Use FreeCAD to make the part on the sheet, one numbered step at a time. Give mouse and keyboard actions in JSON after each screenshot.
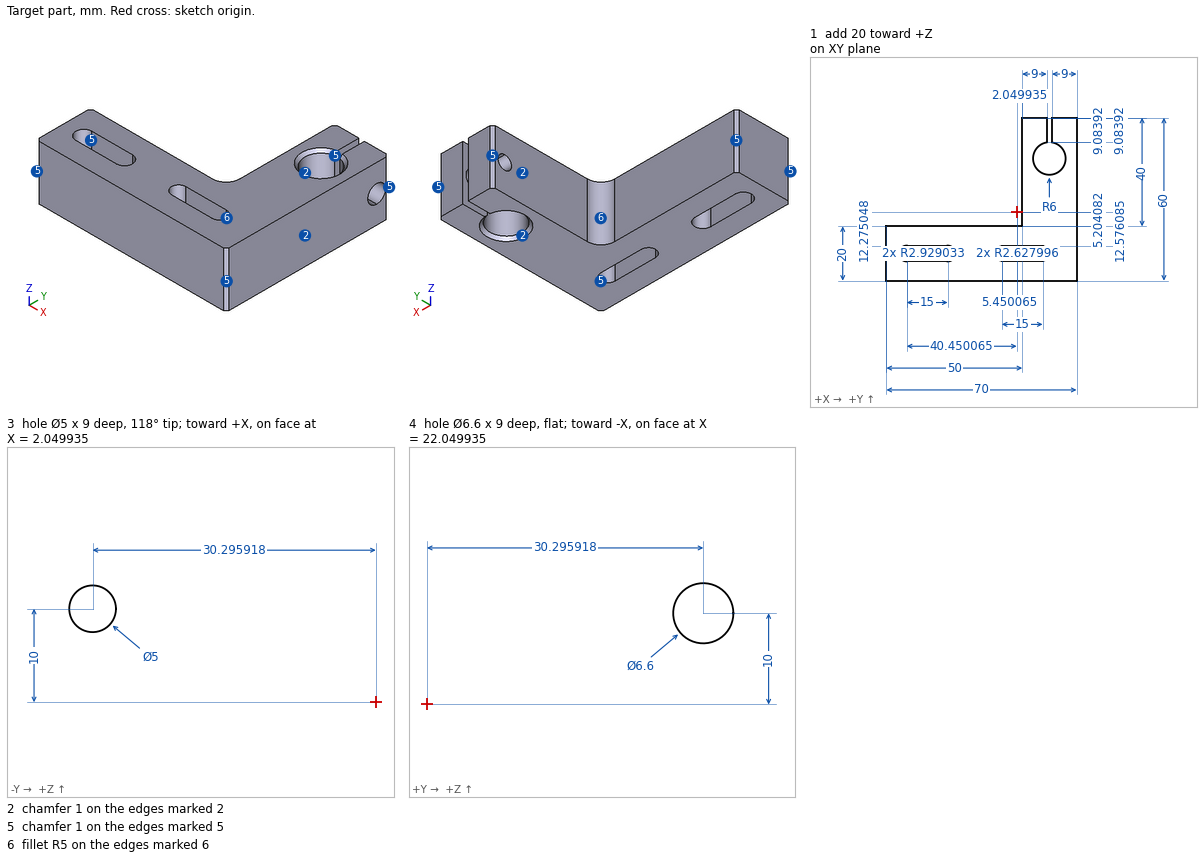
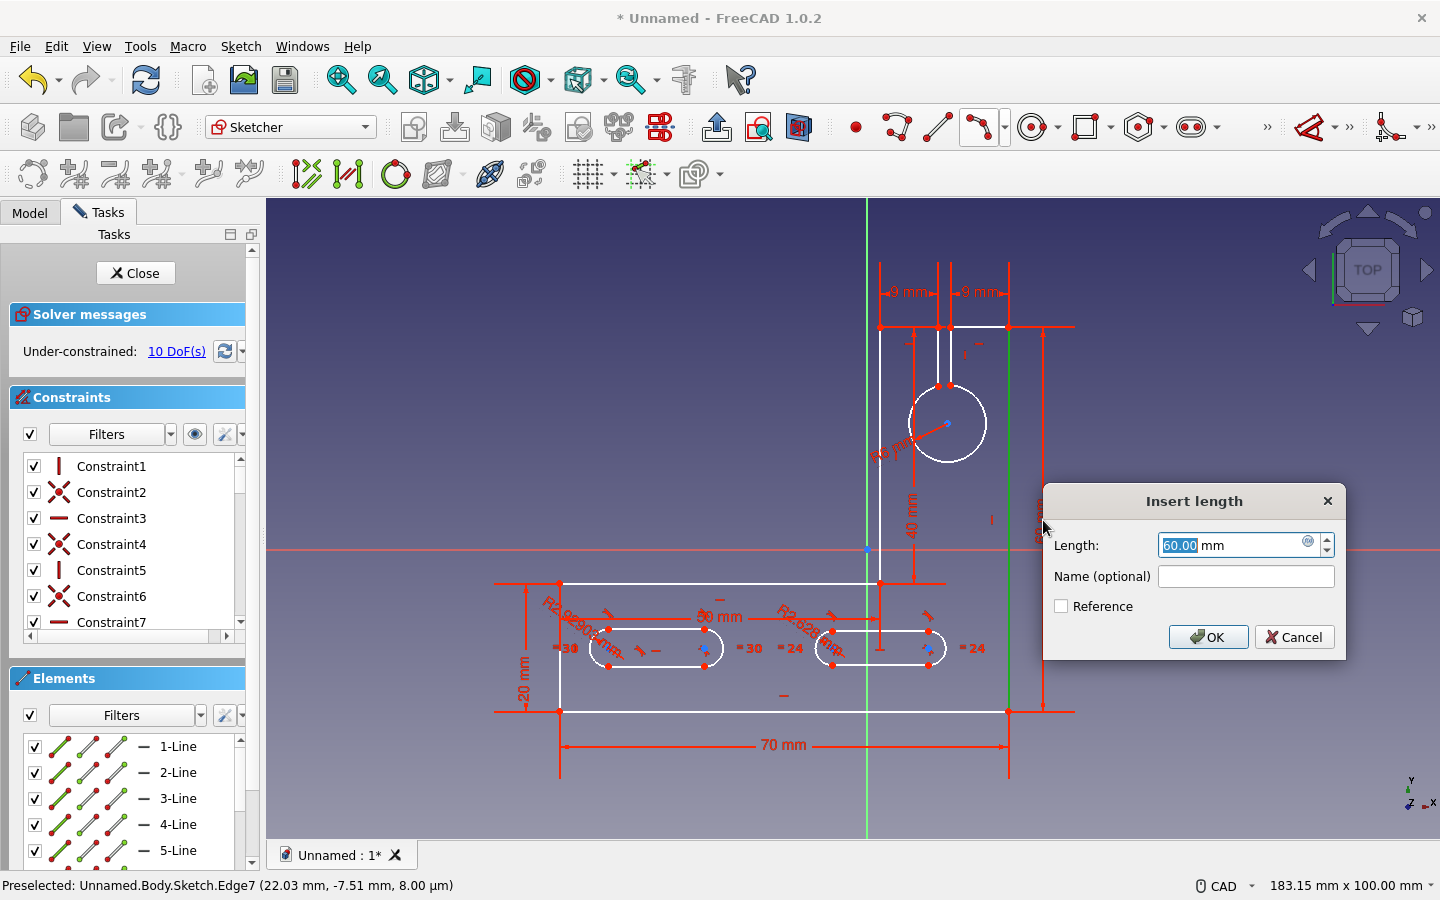
{"action": "type", "text": "60"}
{"action": "key", "text": "Return"}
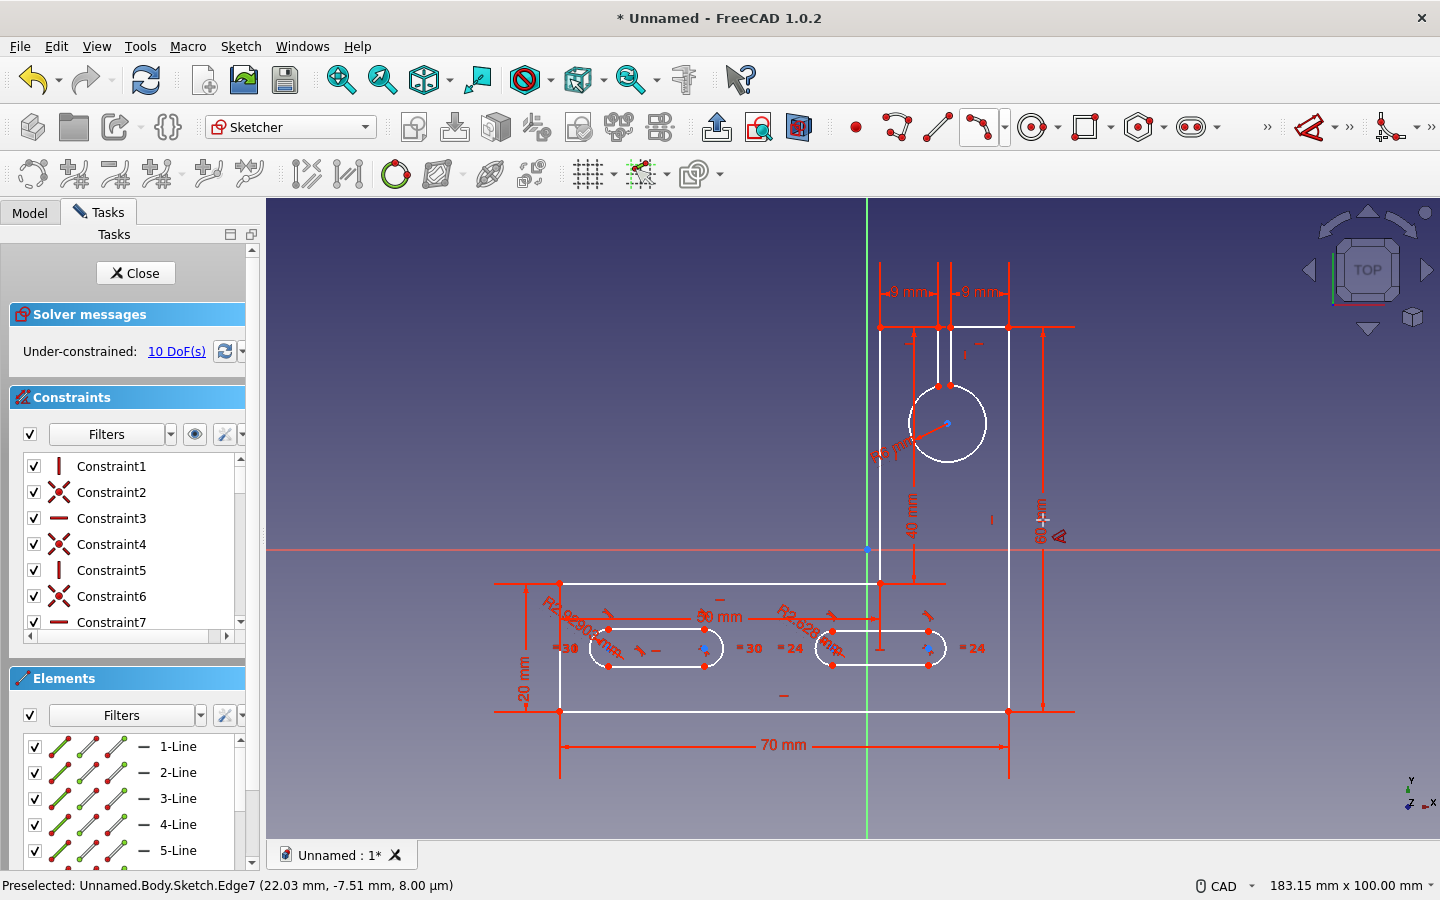
{"action": "left_click", "coordinate": [900, 631]}
{"action": "left_click", "coordinate": [881, 597]}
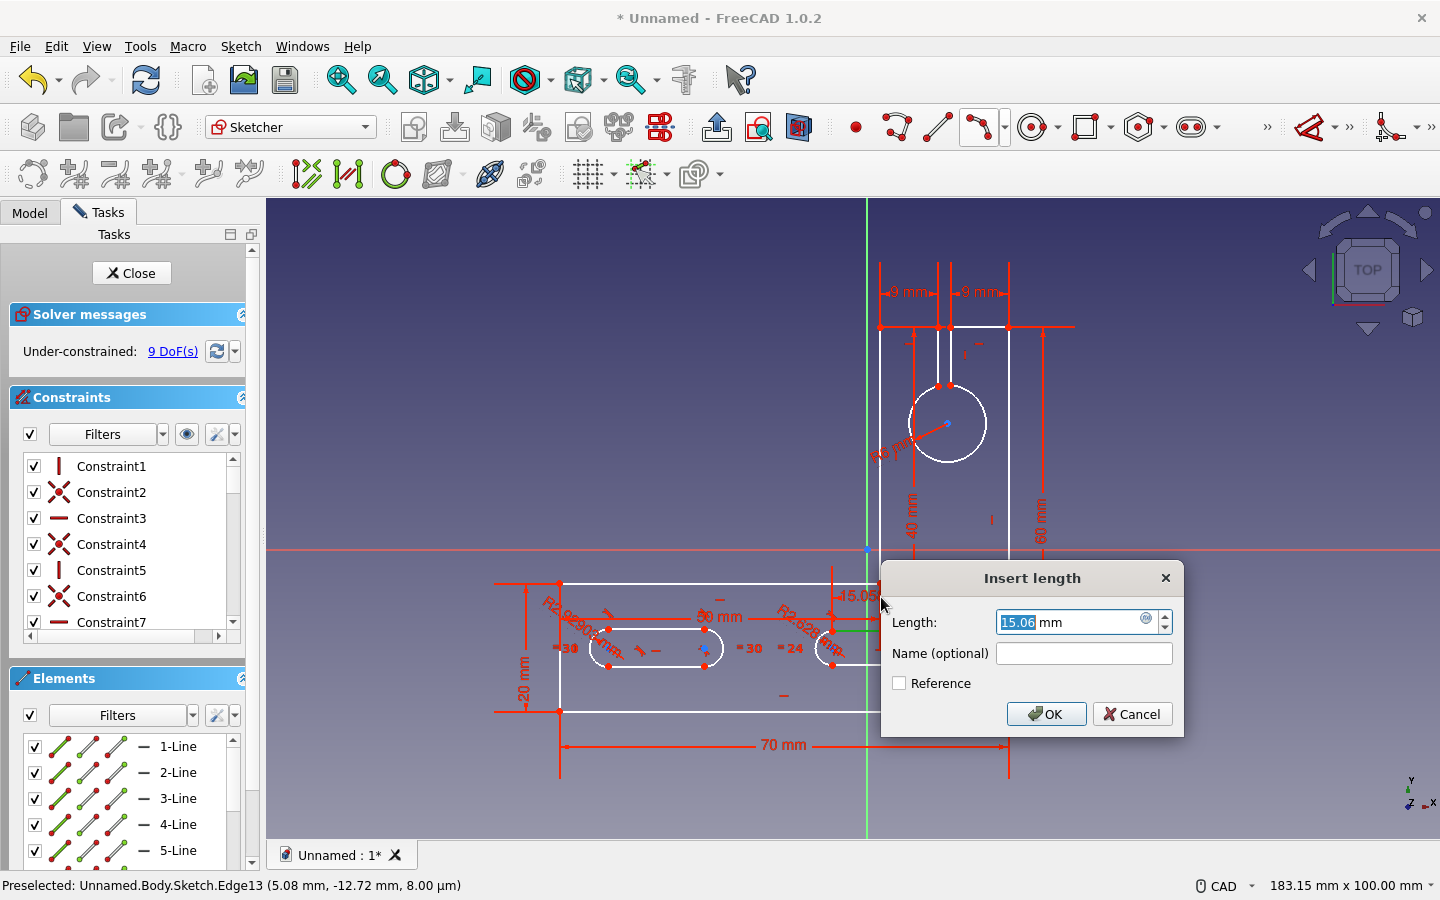
{"action": "type", "text": "15"}
{"action": "key", "text": "Return"}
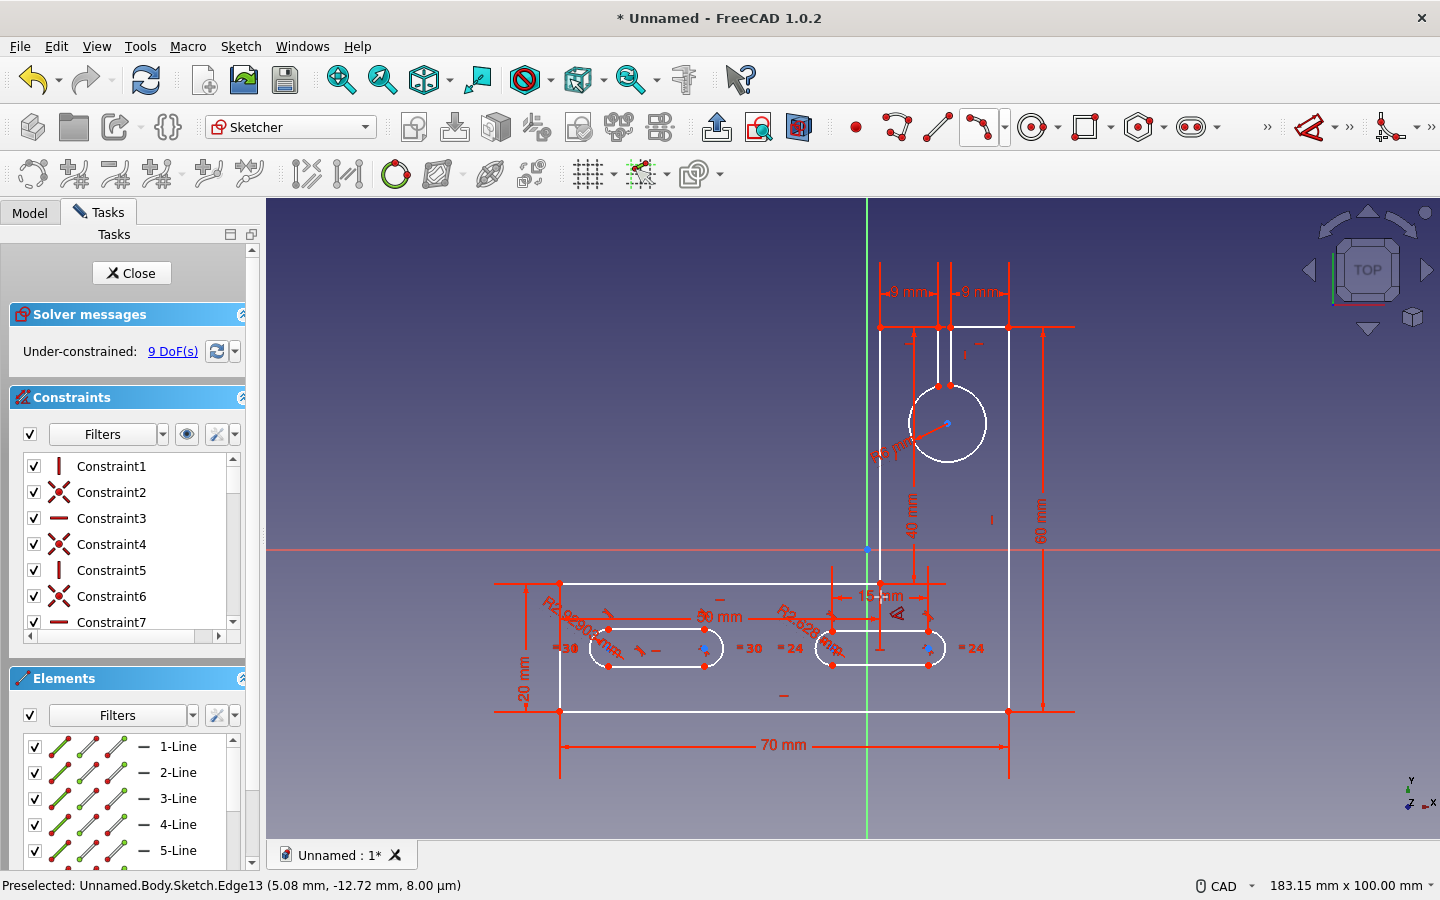
{"action": "left_click", "coordinate": [637, 629]}
{"action": "left_click", "coordinate": [656, 687]}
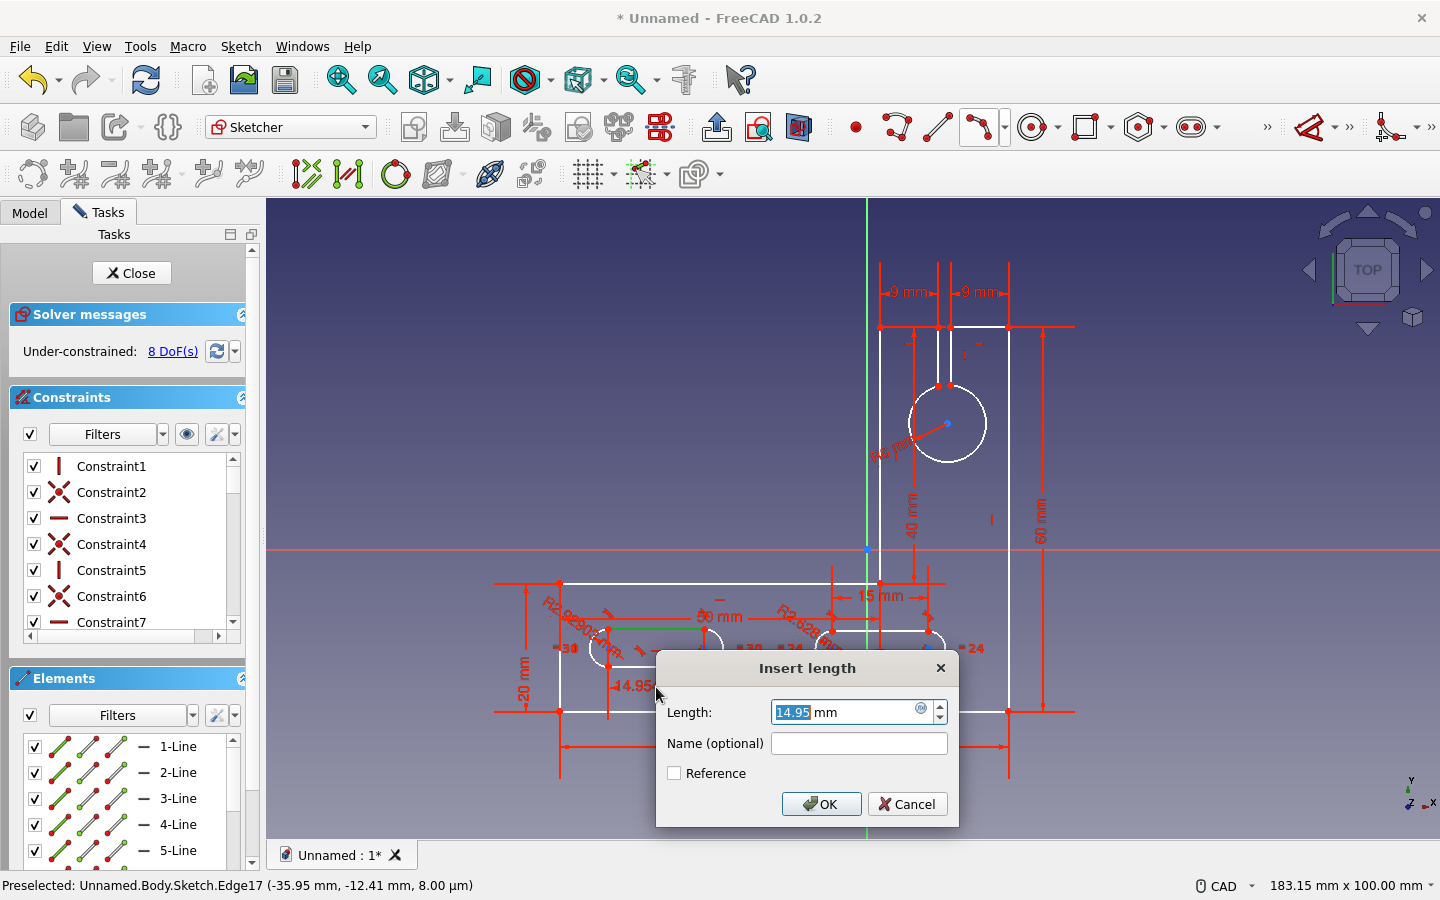
{"action": "type", "text": "15"}
{"action": "key", "text": "Return"}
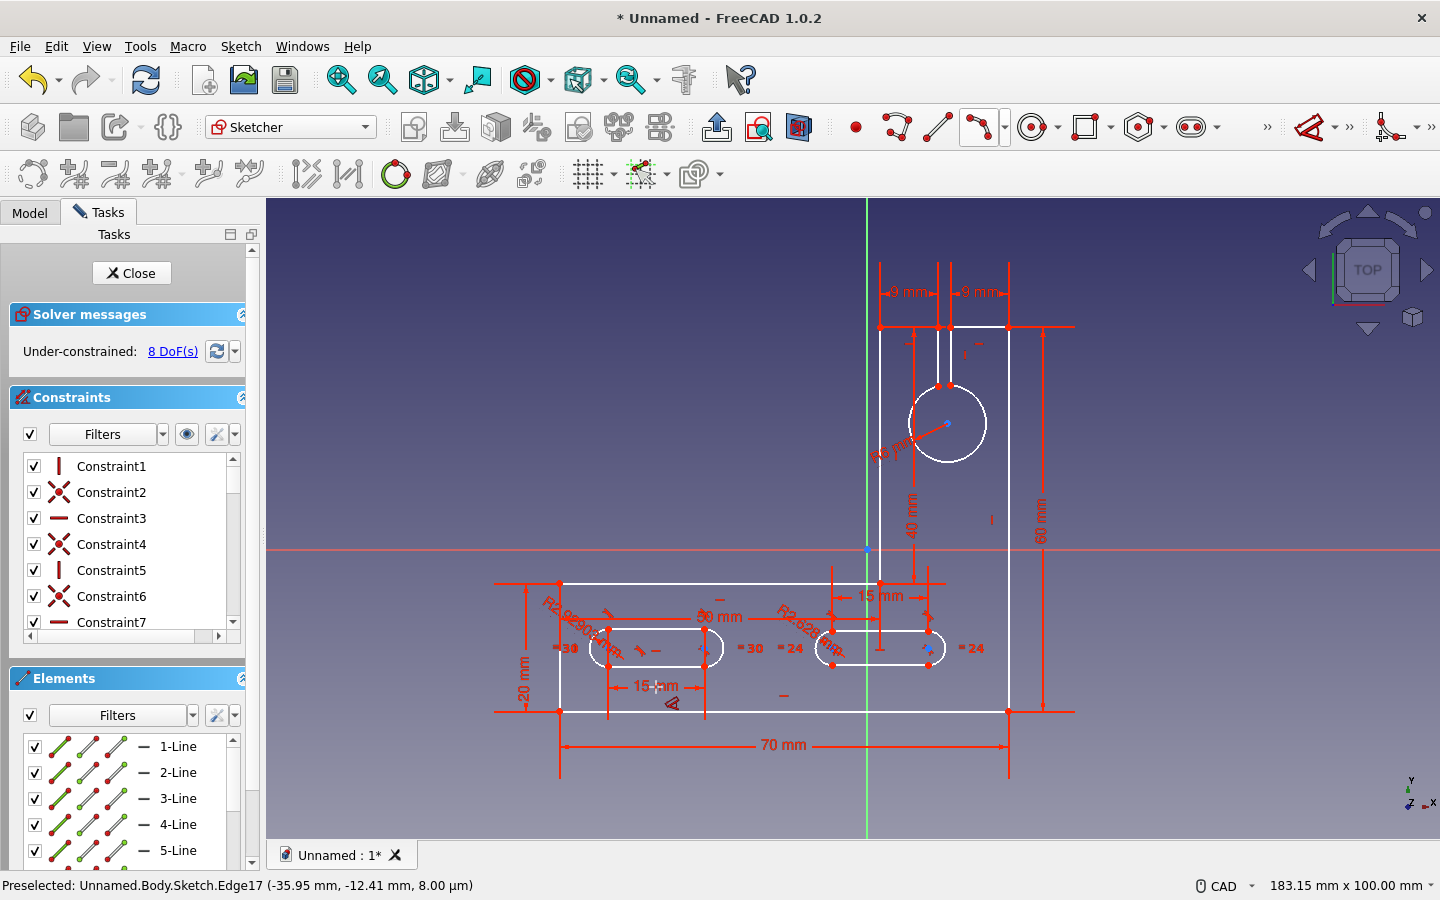
{"action": "left_click", "coordinate": [938, 369]}
{"action": "left_click", "coordinate": [972, 357]}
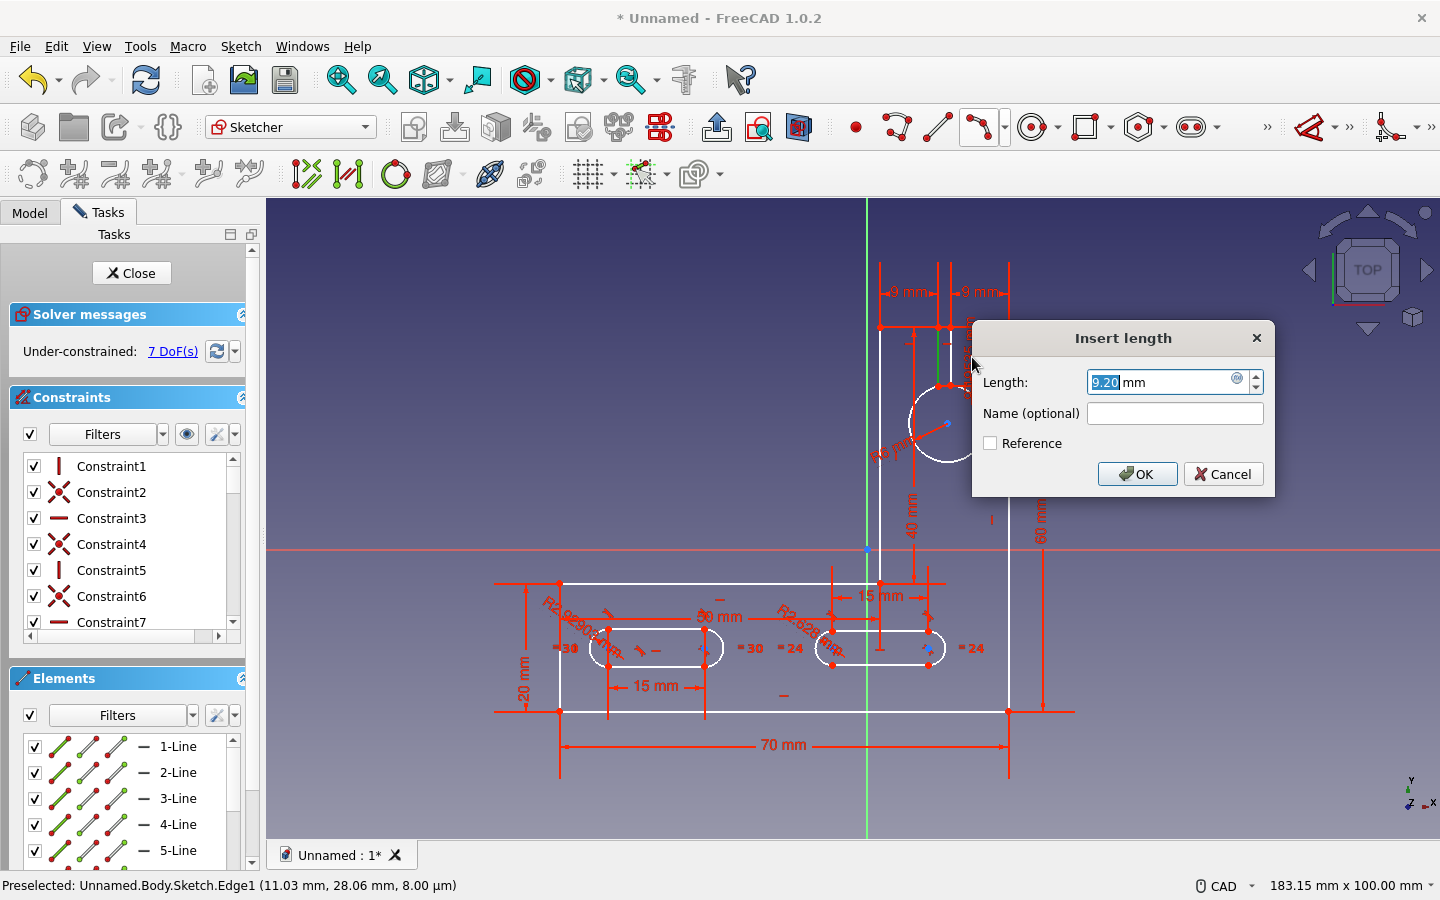
{"action": "type", "text": "9.08392"}
{"action": "key", "text": "Return"}